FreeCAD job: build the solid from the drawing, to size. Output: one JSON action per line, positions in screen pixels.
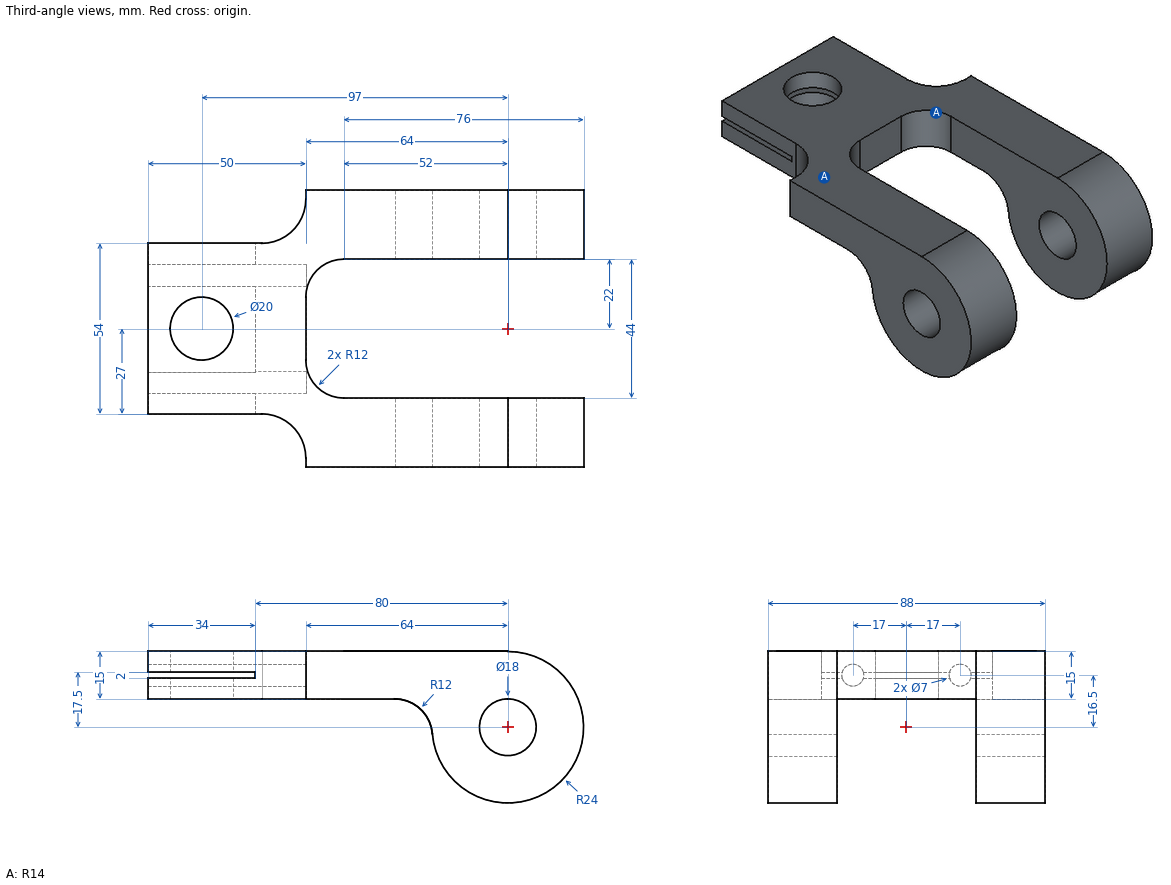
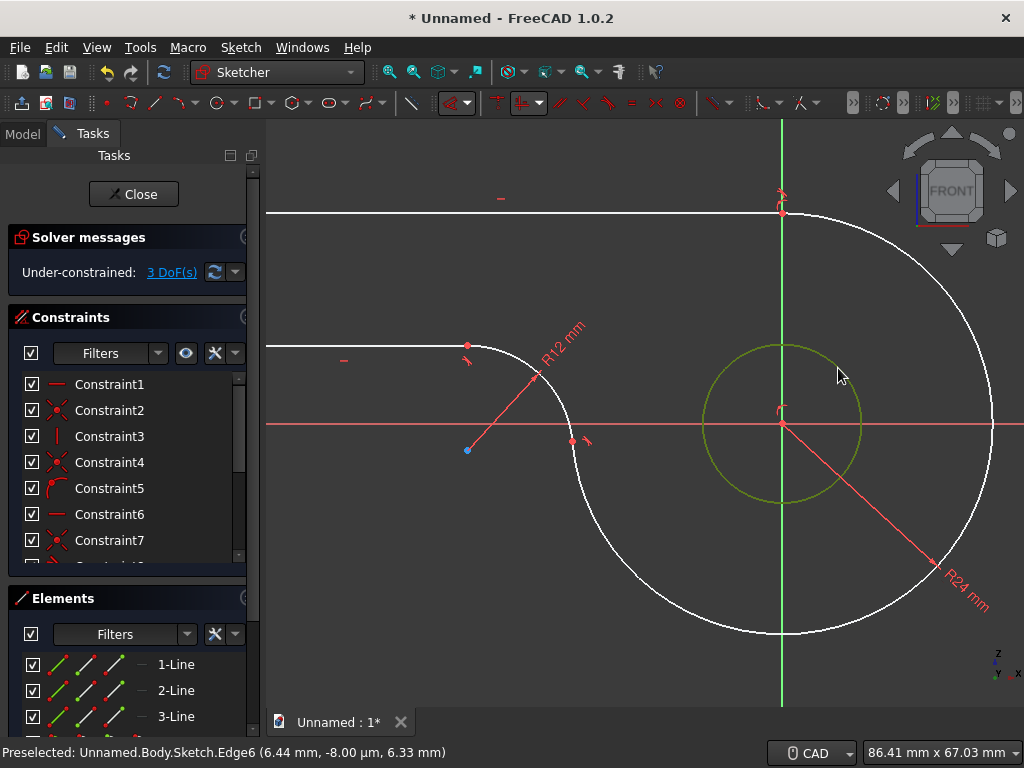
{"action": "key", "text": "k o"}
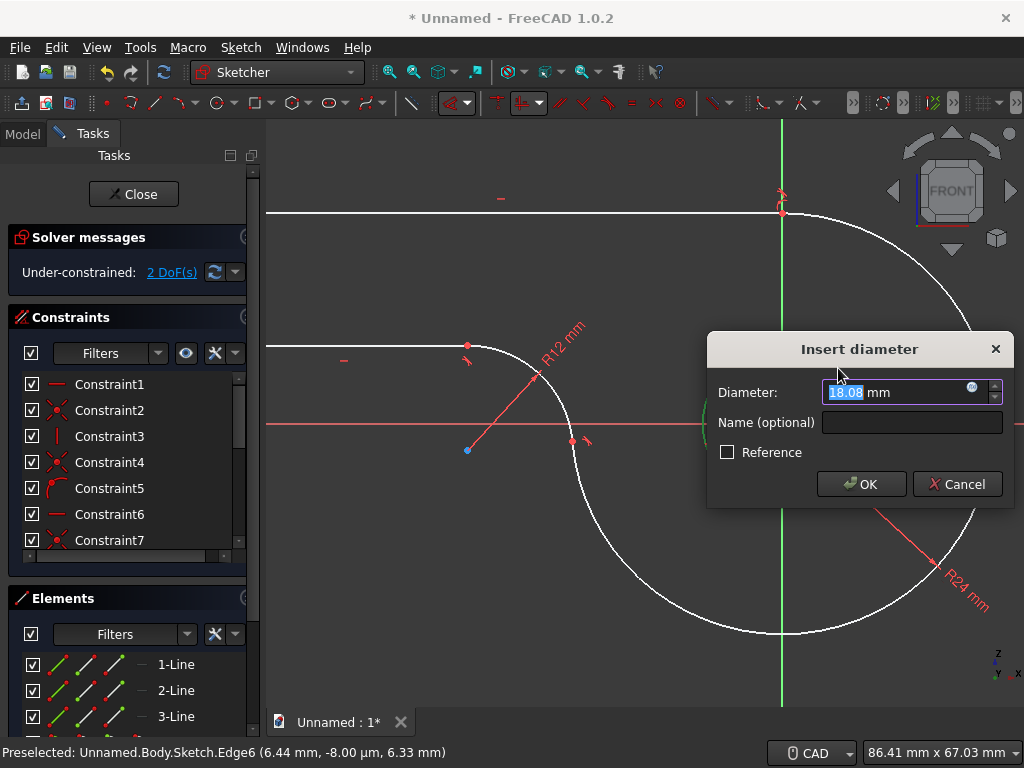
{"action": "type", "text": "18"}
{"action": "key", "text": "Return"}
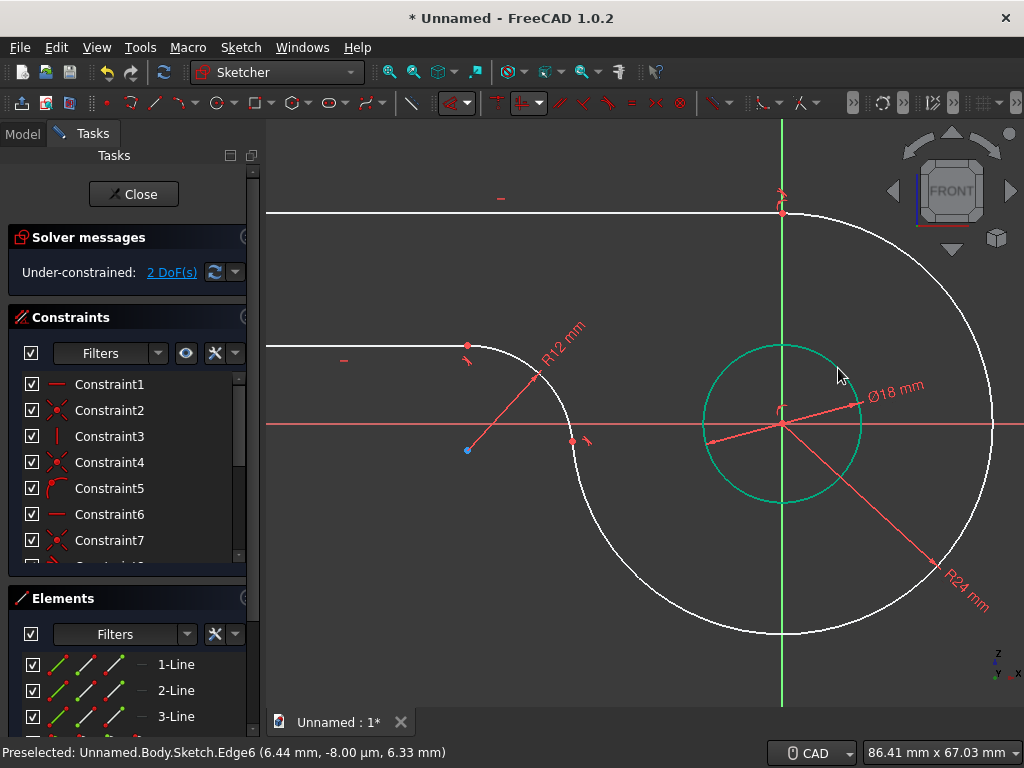
{"action": "scroll", "coordinate": [573, 441], "scroll_direction": "down", "scroll_amount": 3}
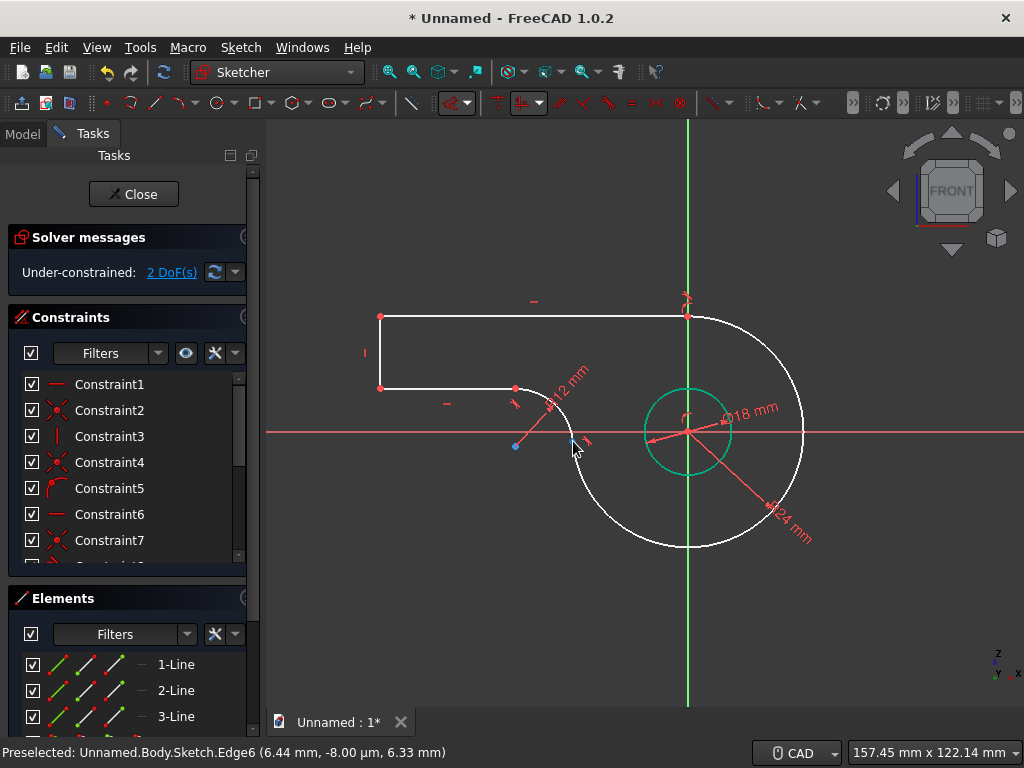
{"action": "left_click", "coordinate": [380, 367]}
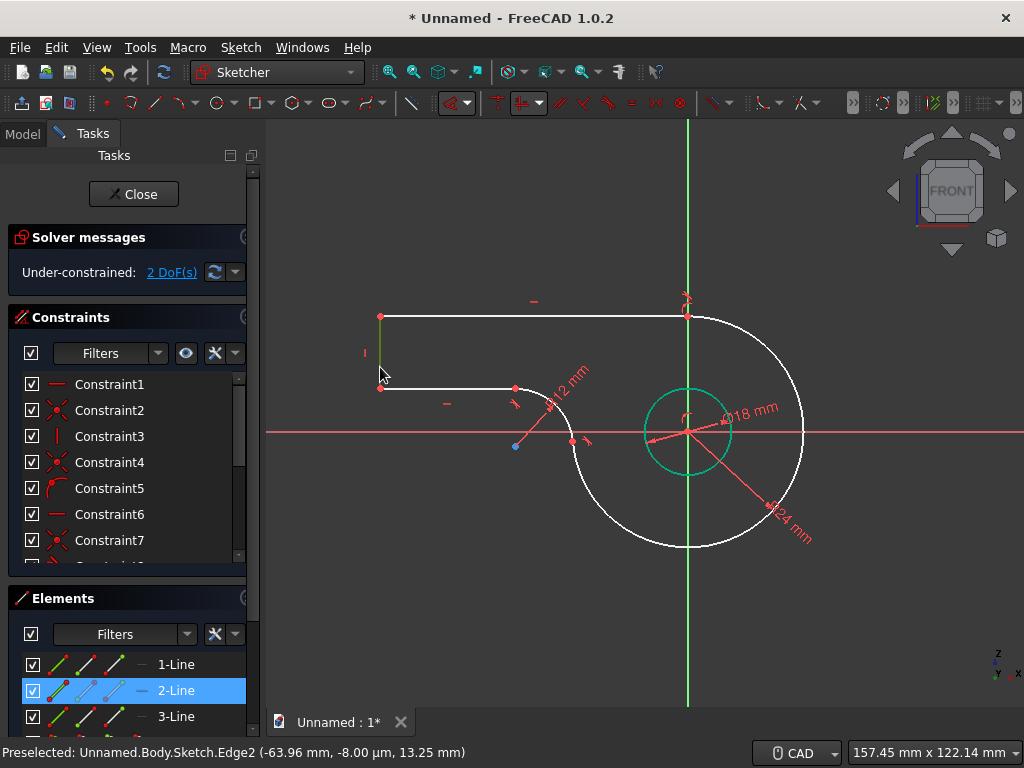
{"action": "left_click", "coordinate": [470, 104]}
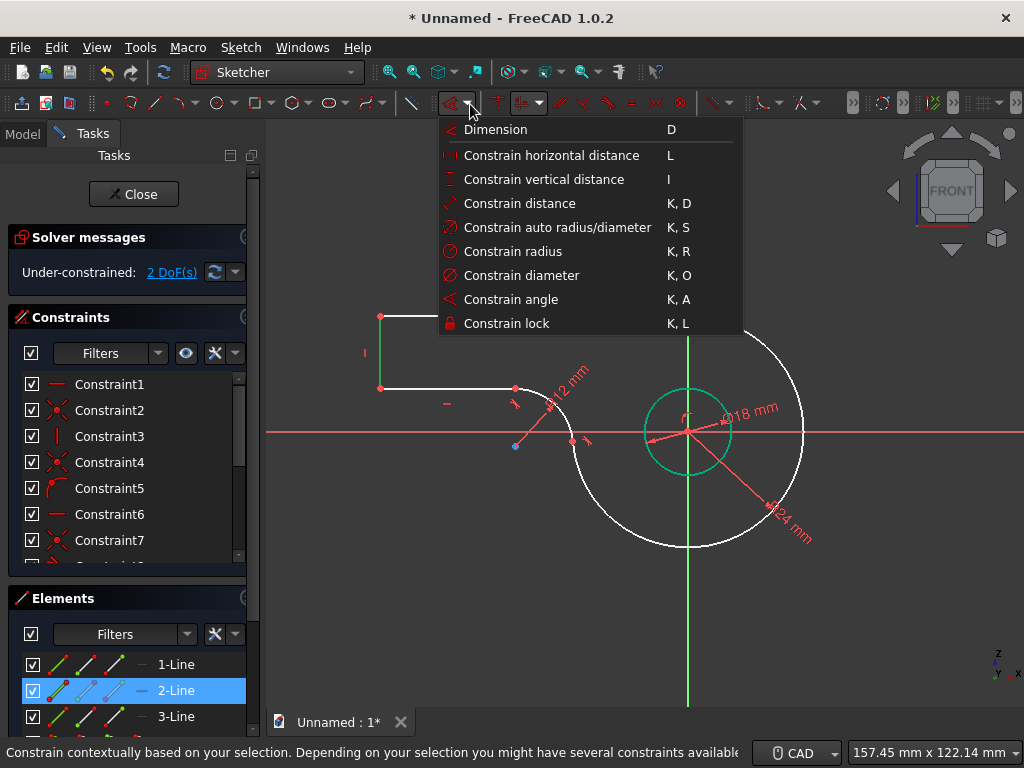
{"action": "left_click", "coordinate": [591, 179]}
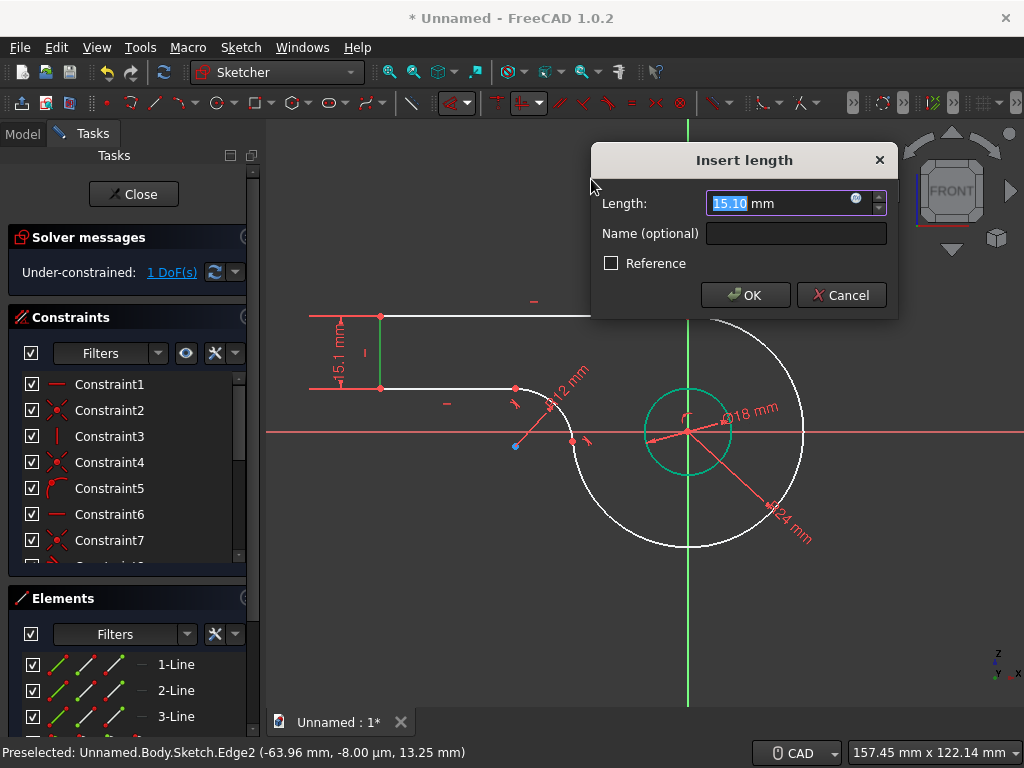
{"action": "type", "text": "15"}
{"action": "key", "text": "Return"}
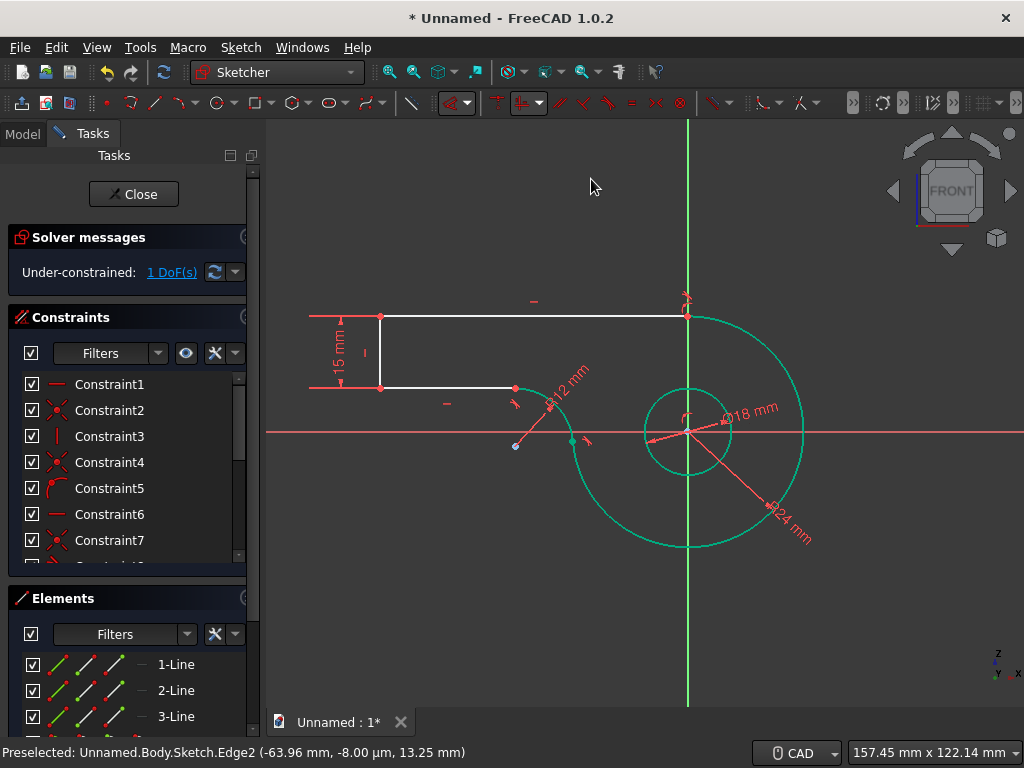
{"action": "left_click", "coordinate": [472, 316]}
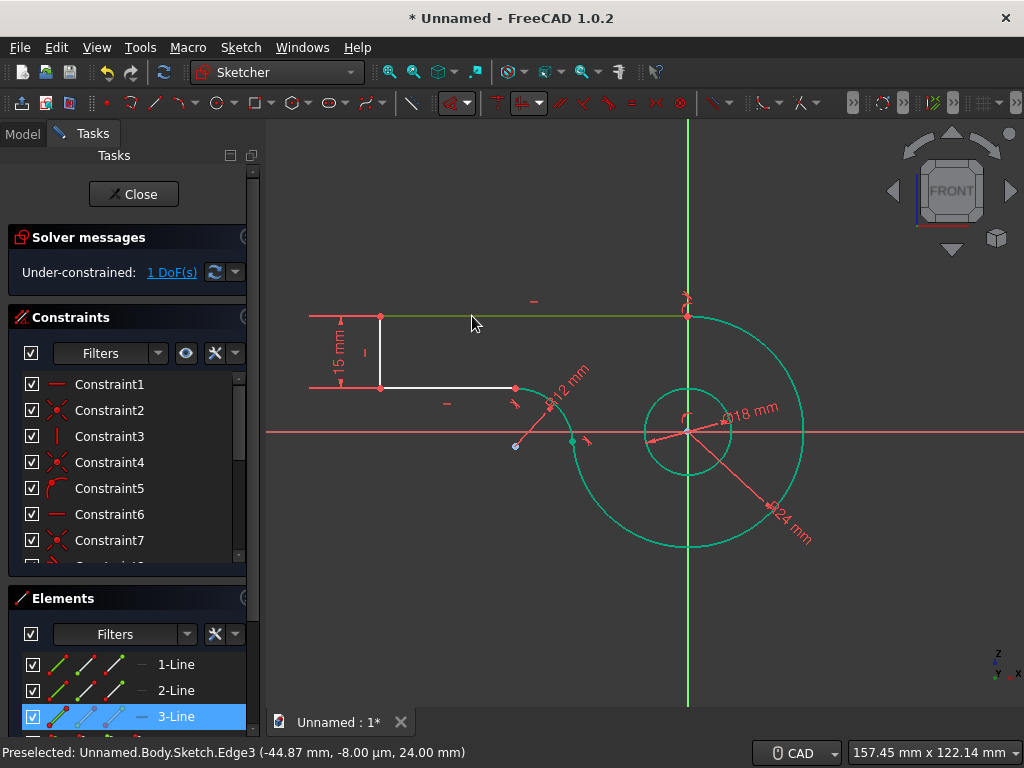
{"action": "key", "text": "l"}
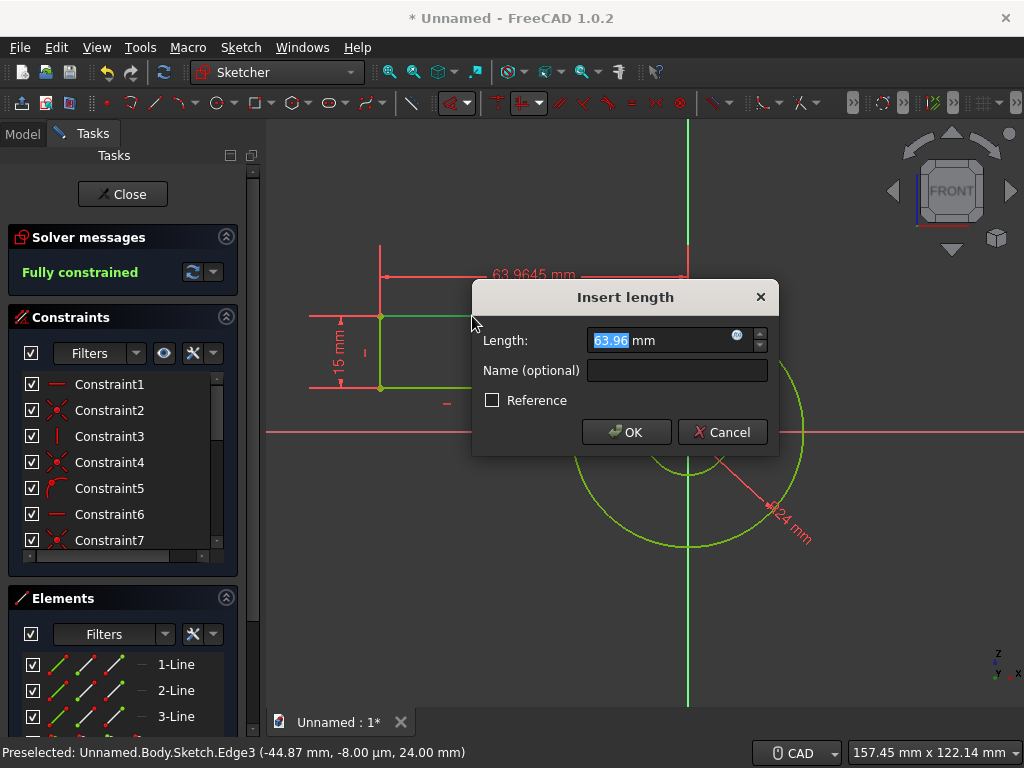
{"action": "type", "text": "64"}
{"action": "key", "text": "Return"}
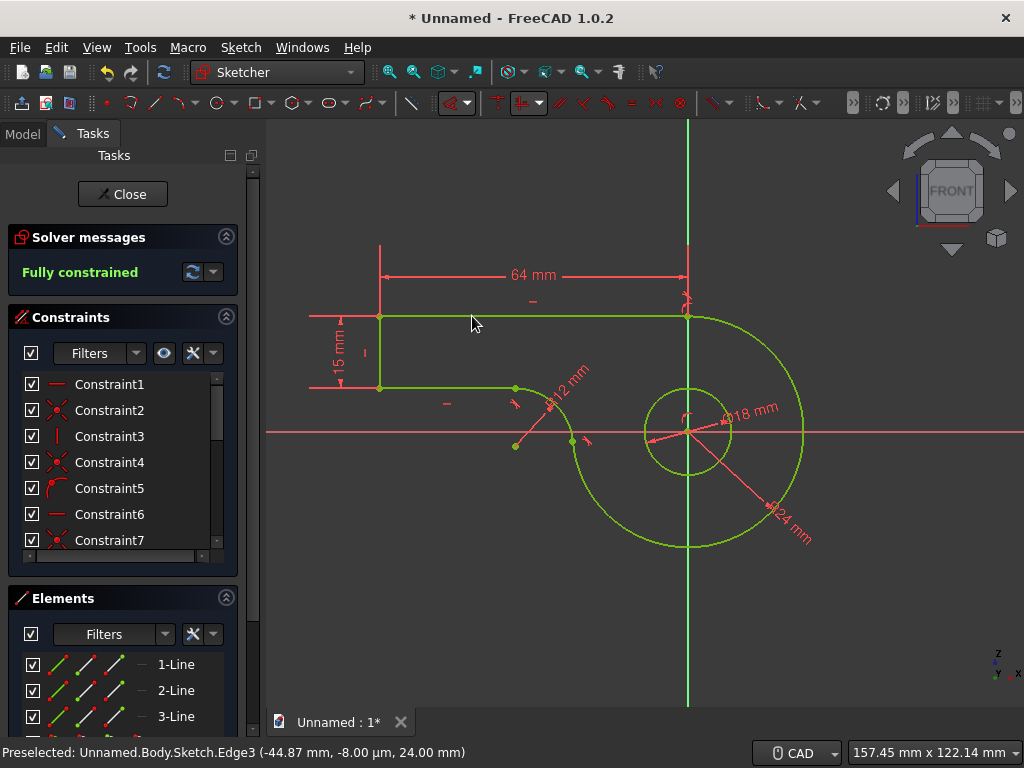
{"action": "left_click", "coordinate": [123, 194]}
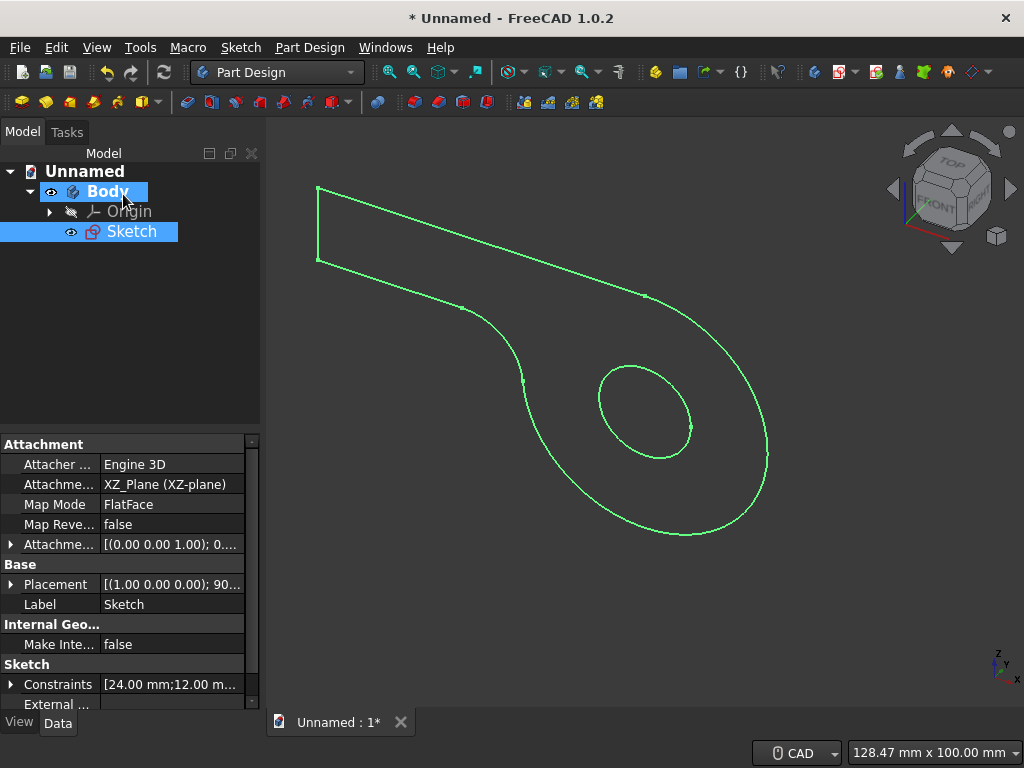
{"action": "left_click", "coordinate": [22, 102]}